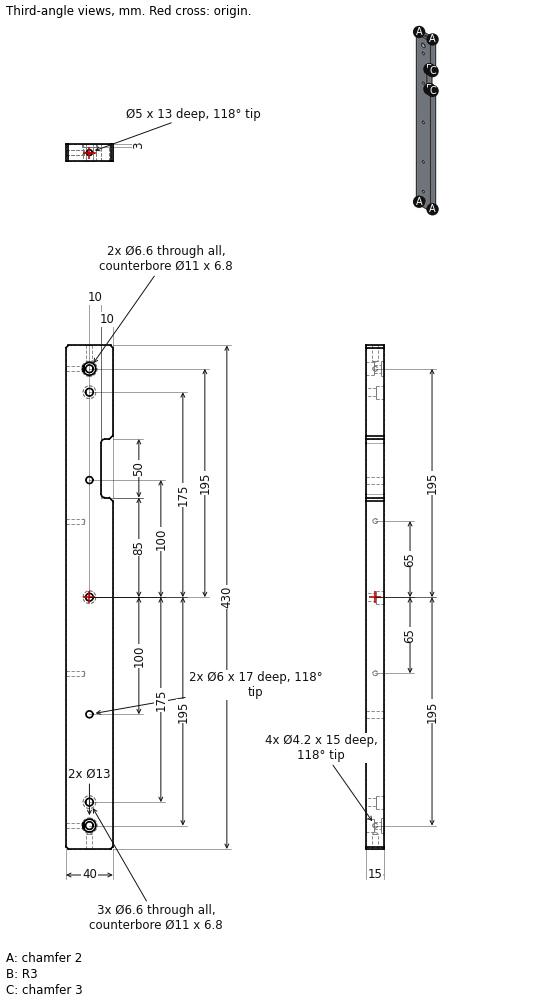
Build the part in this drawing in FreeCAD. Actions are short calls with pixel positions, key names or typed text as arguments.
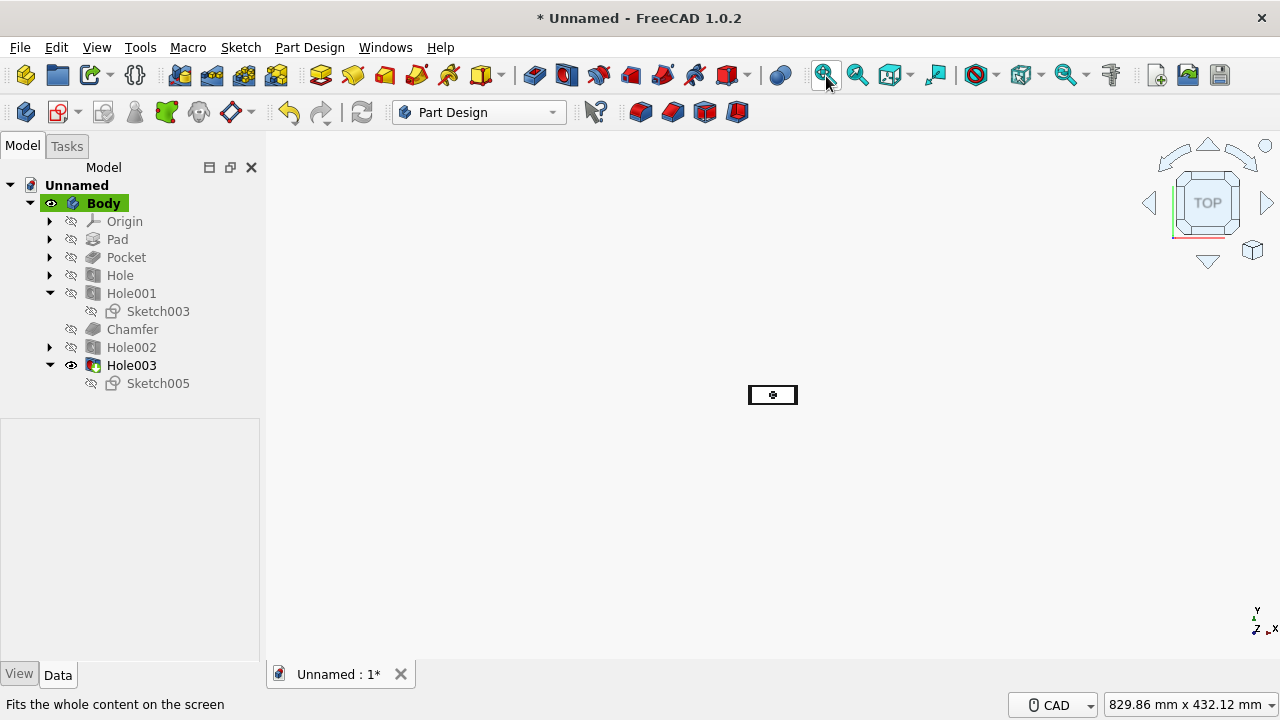
key(5)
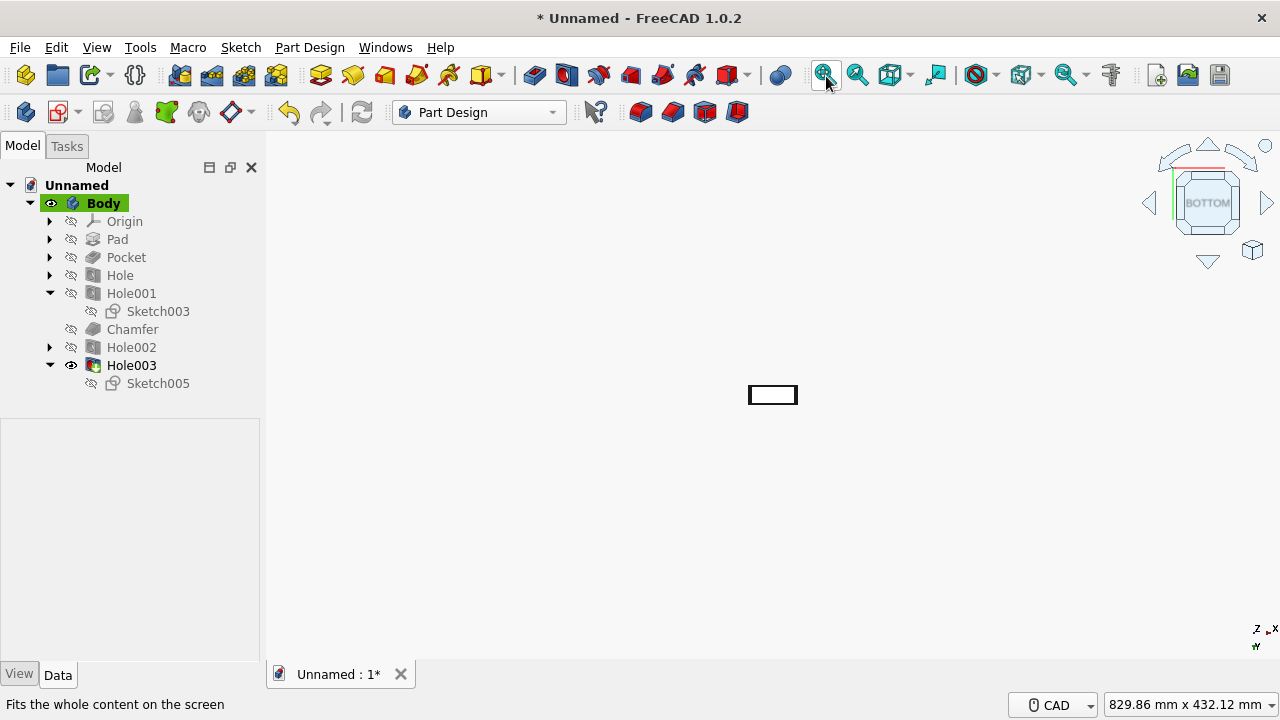
click(826, 76)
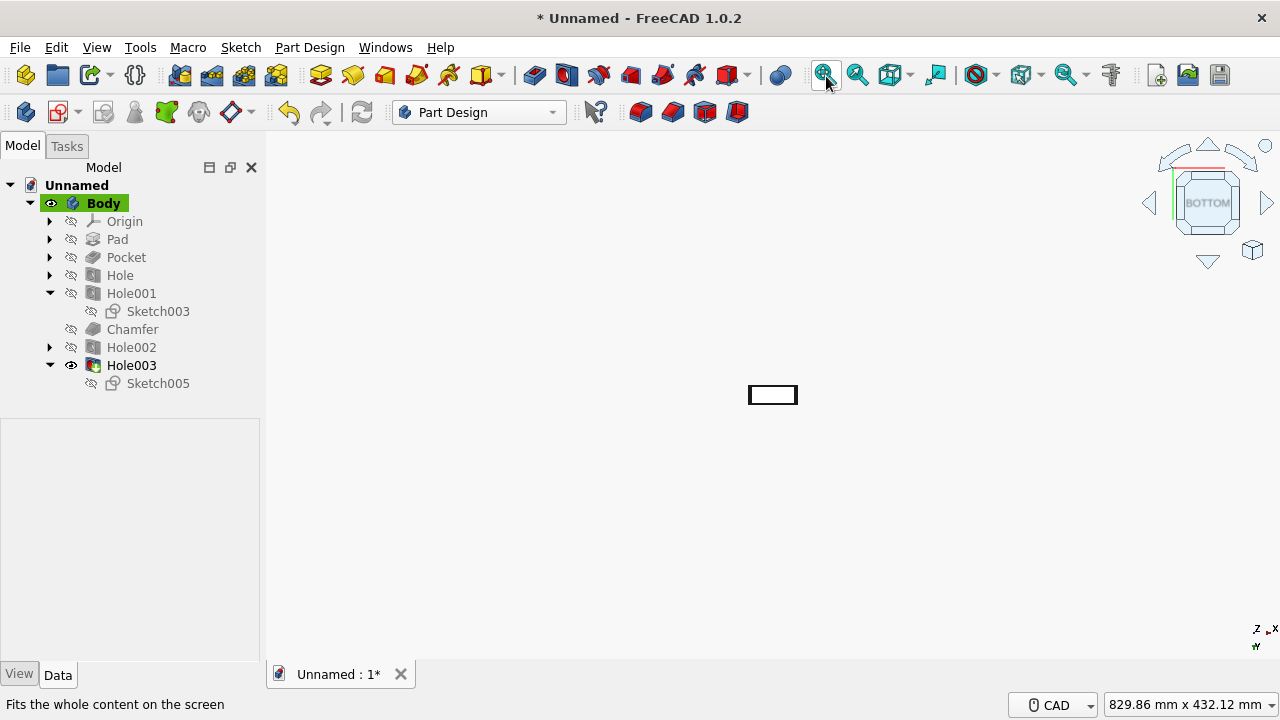
click(786, 394)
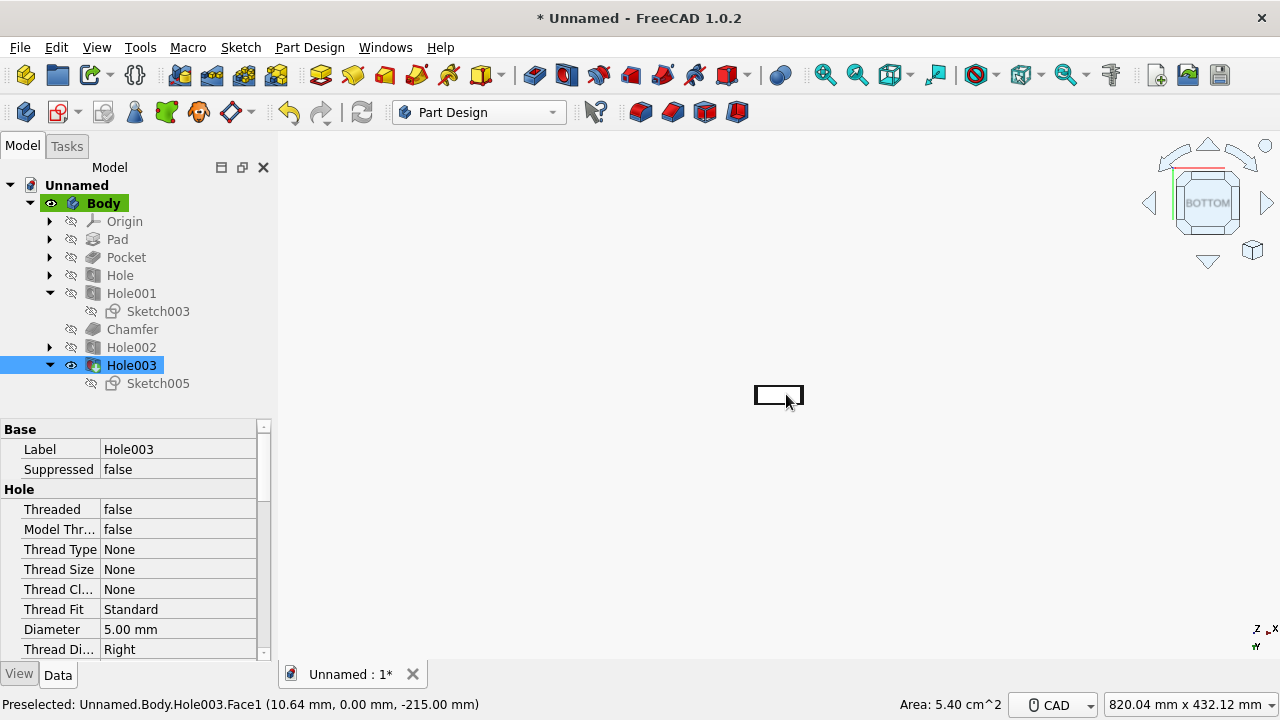
click(58, 112)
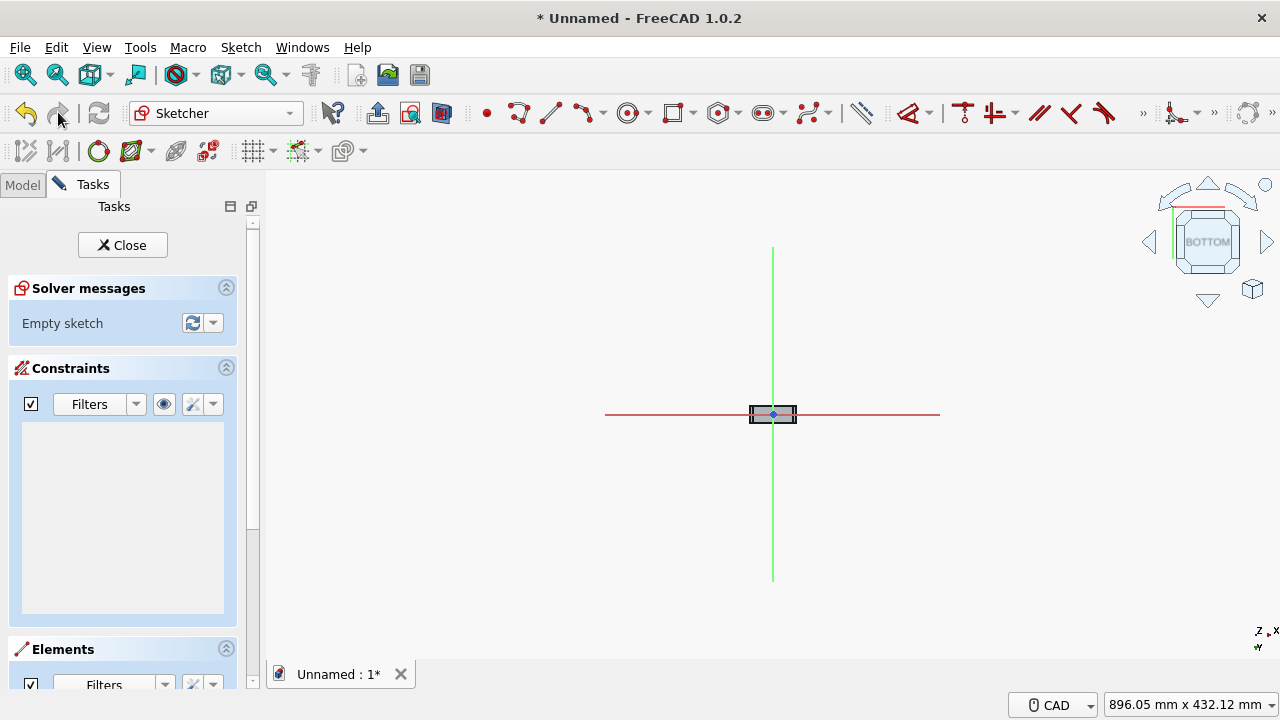
scroll(777, 414, up, 15)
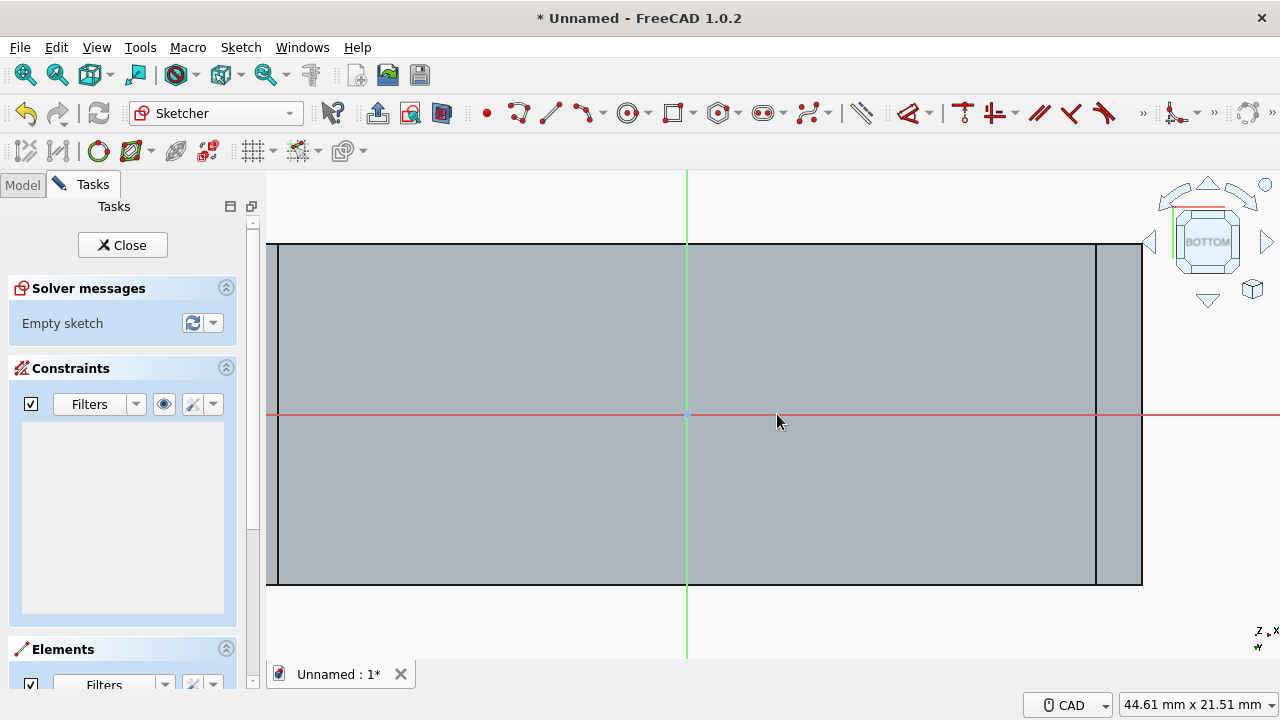
scroll(677, 414, up, 5)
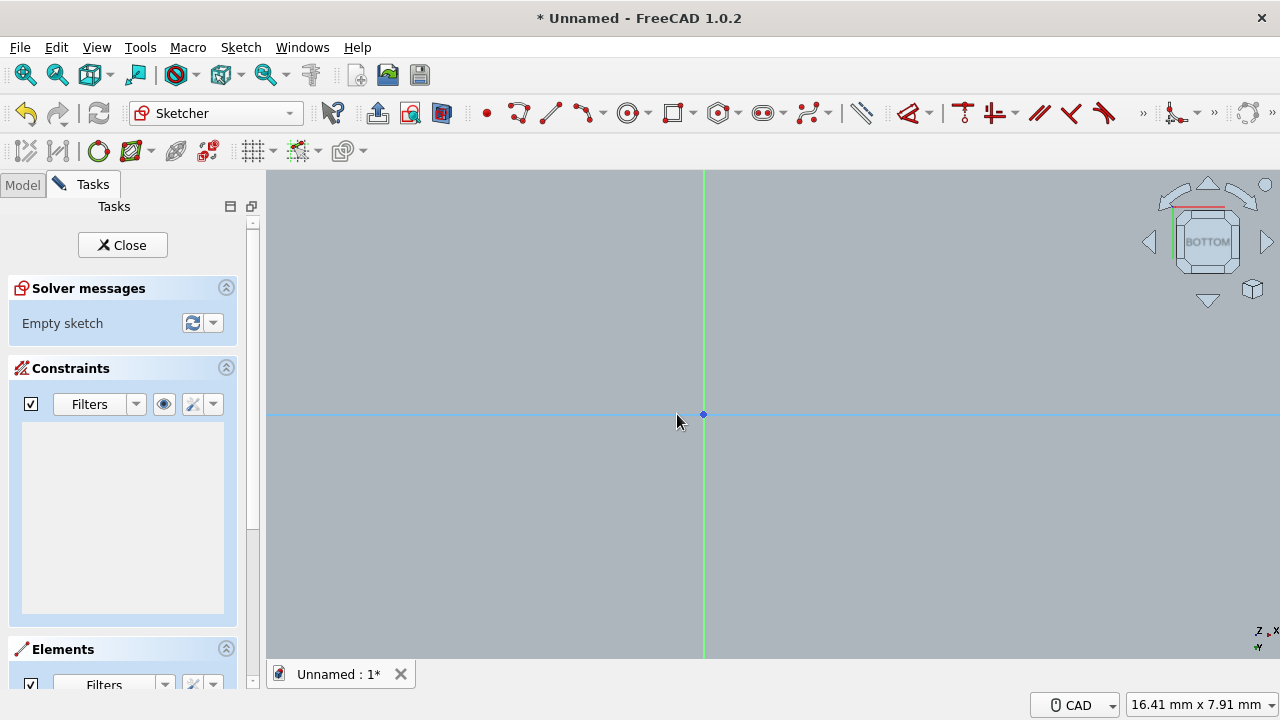
click(628, 114)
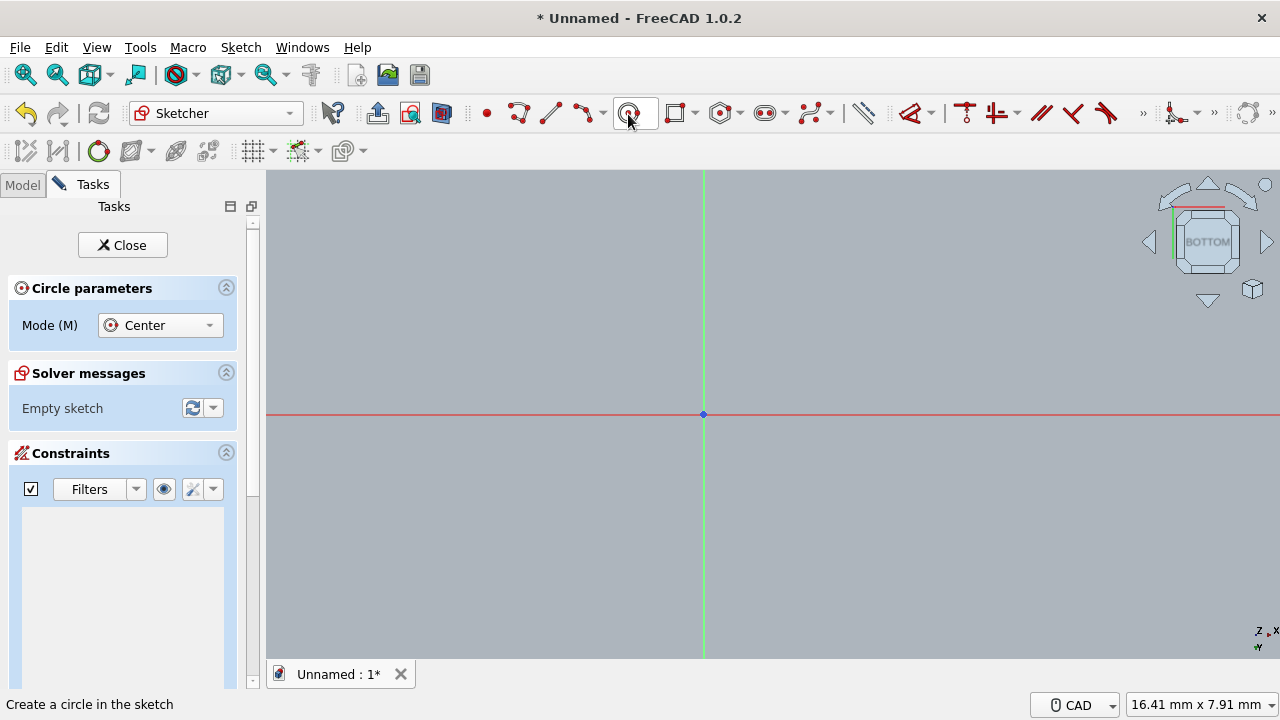
click(704, 414)
move(813, 305)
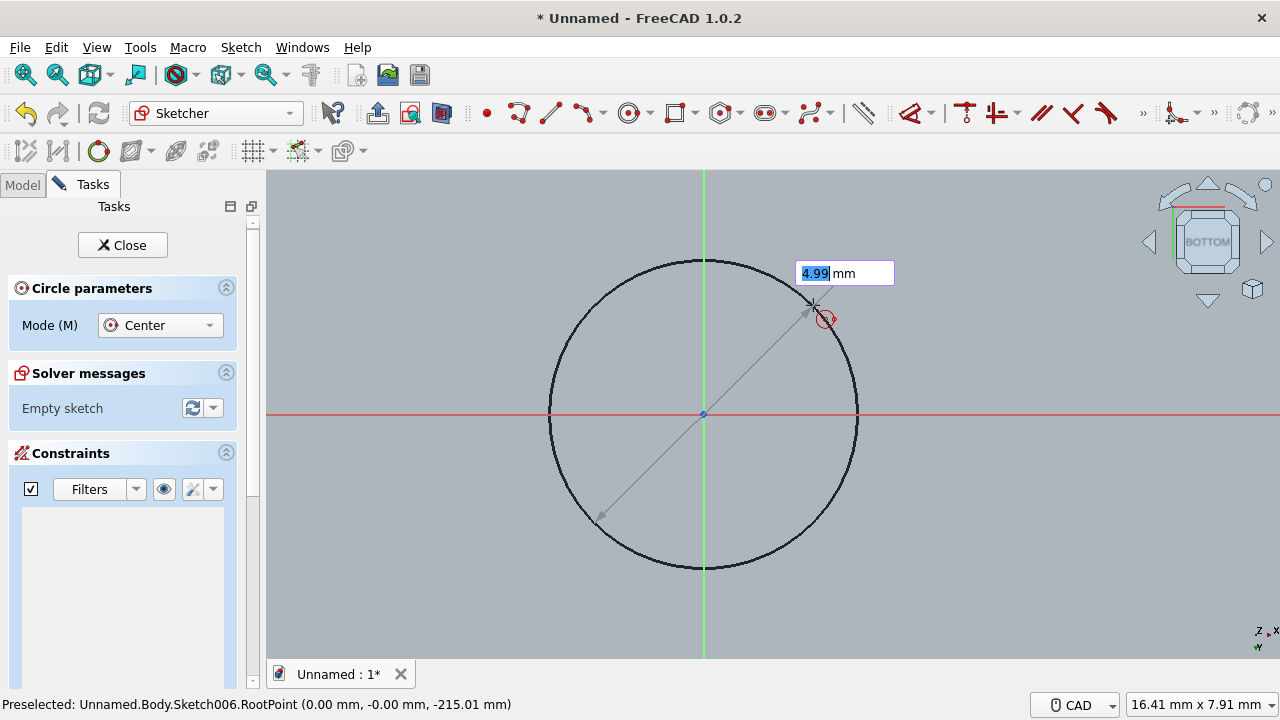
text(5)
key(Return)
key(Escape)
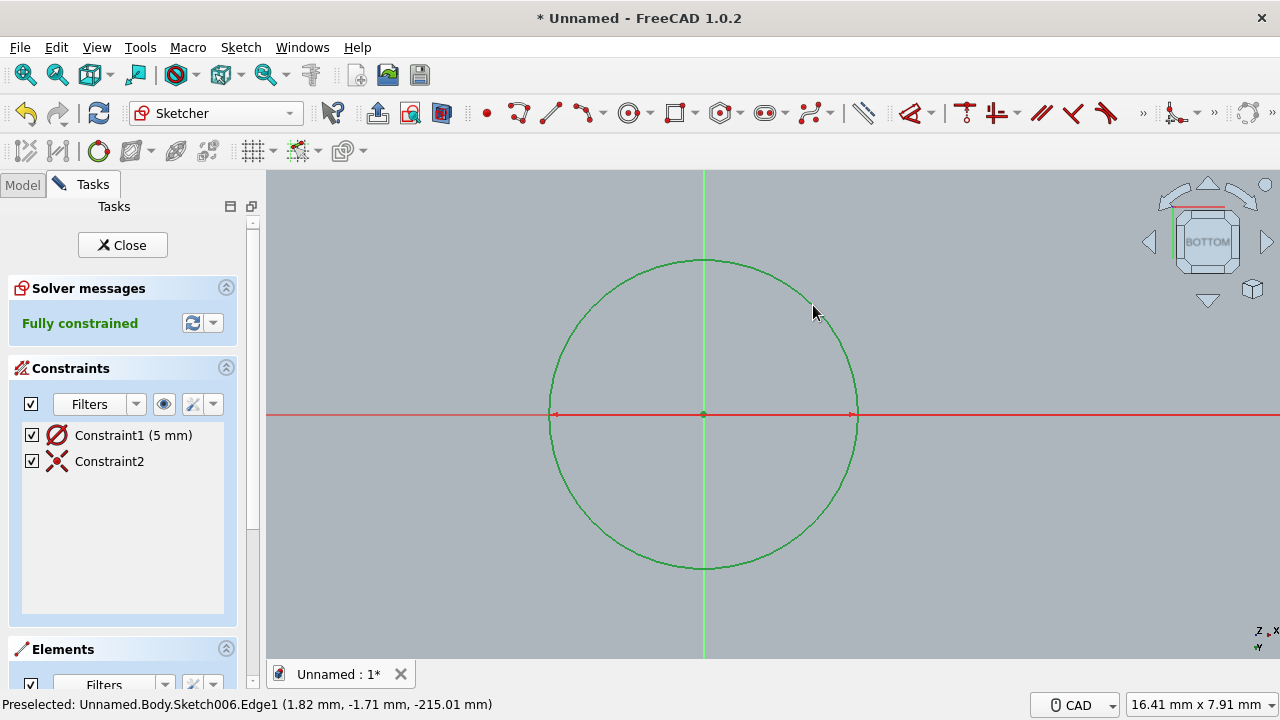
click(123, 245)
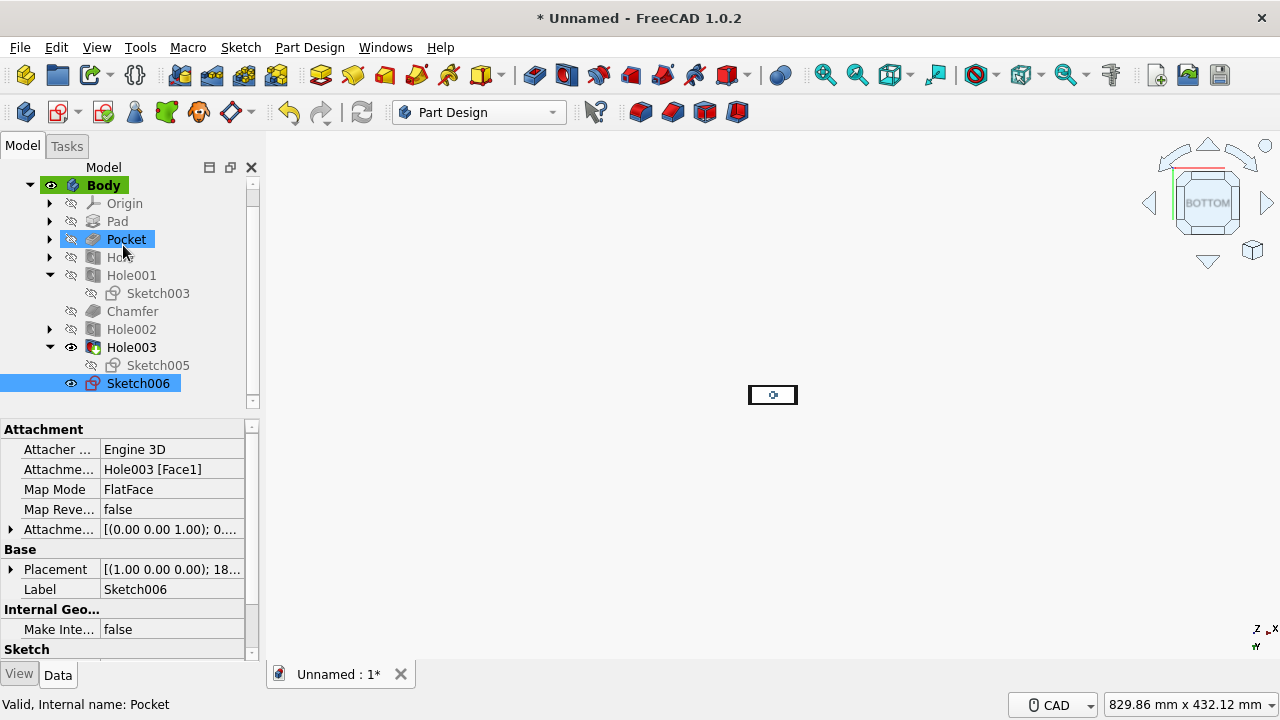
click(568, 76)